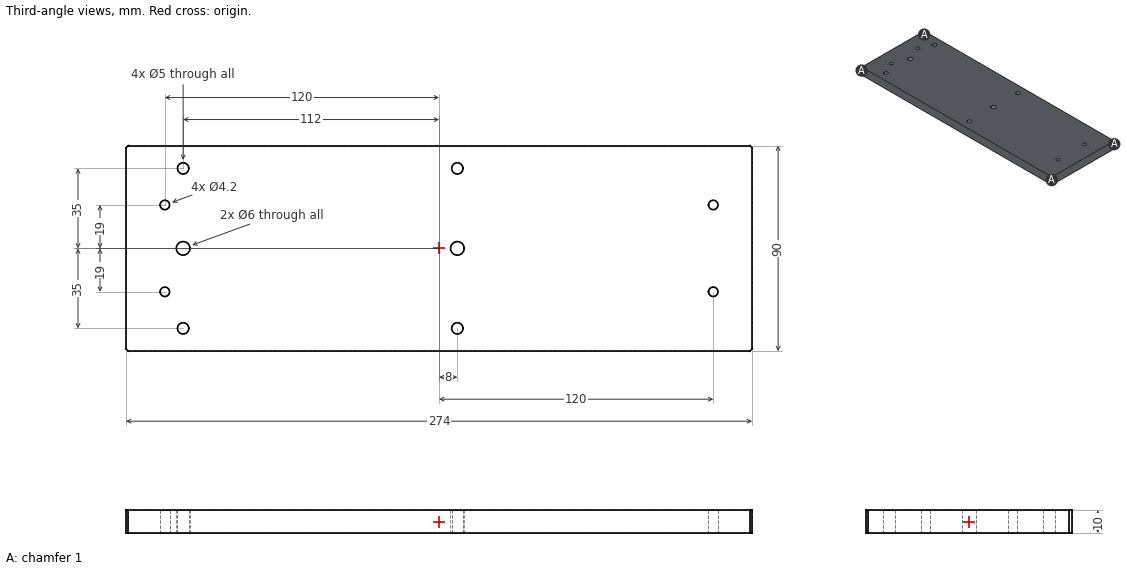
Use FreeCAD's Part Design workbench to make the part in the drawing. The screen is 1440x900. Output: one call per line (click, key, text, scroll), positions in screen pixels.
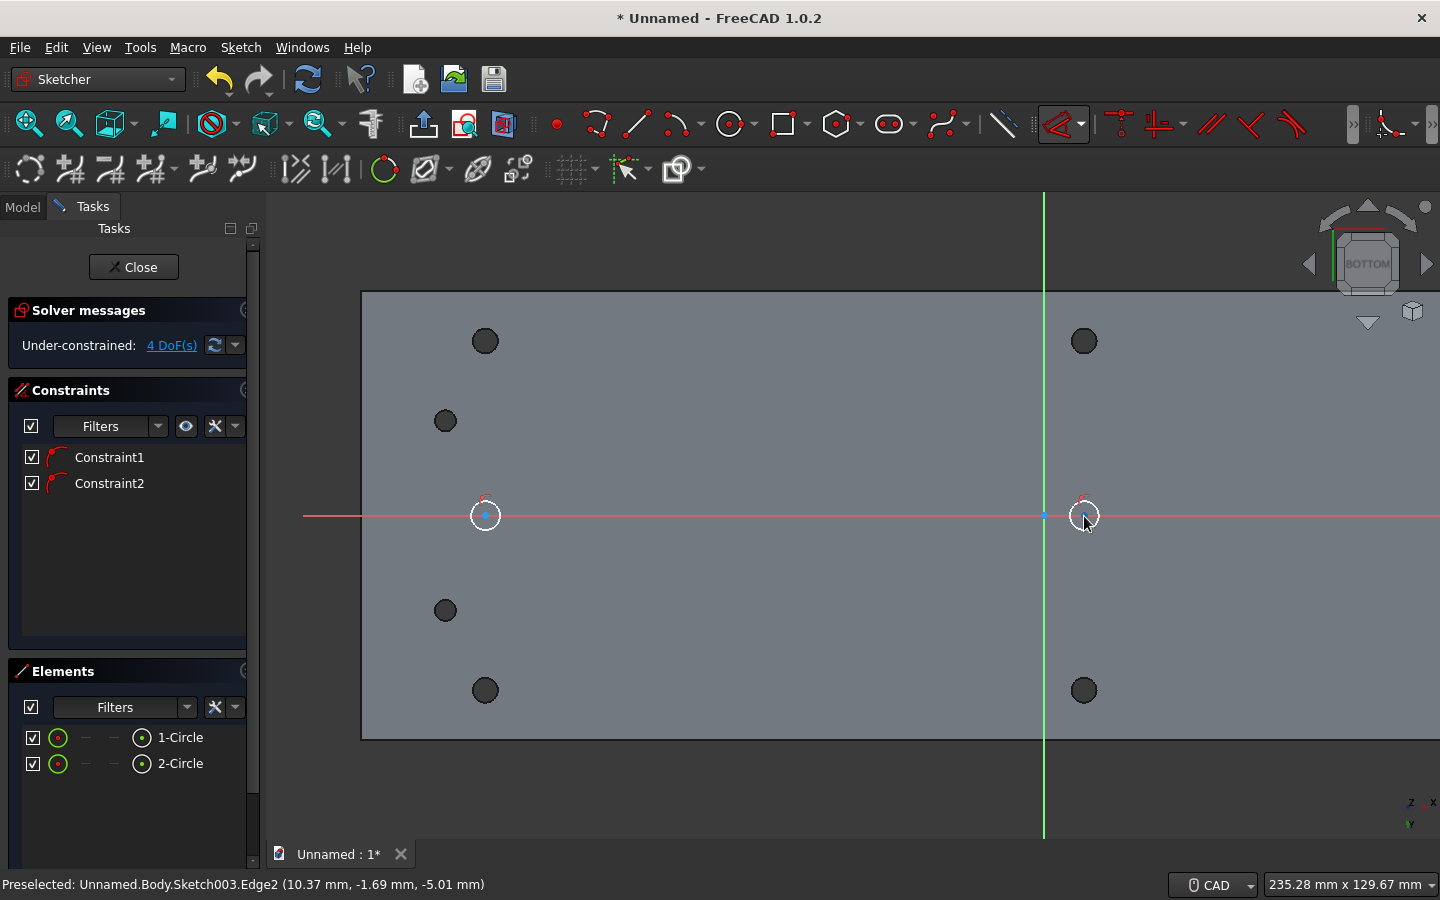
scroll(496, 505, up, 2)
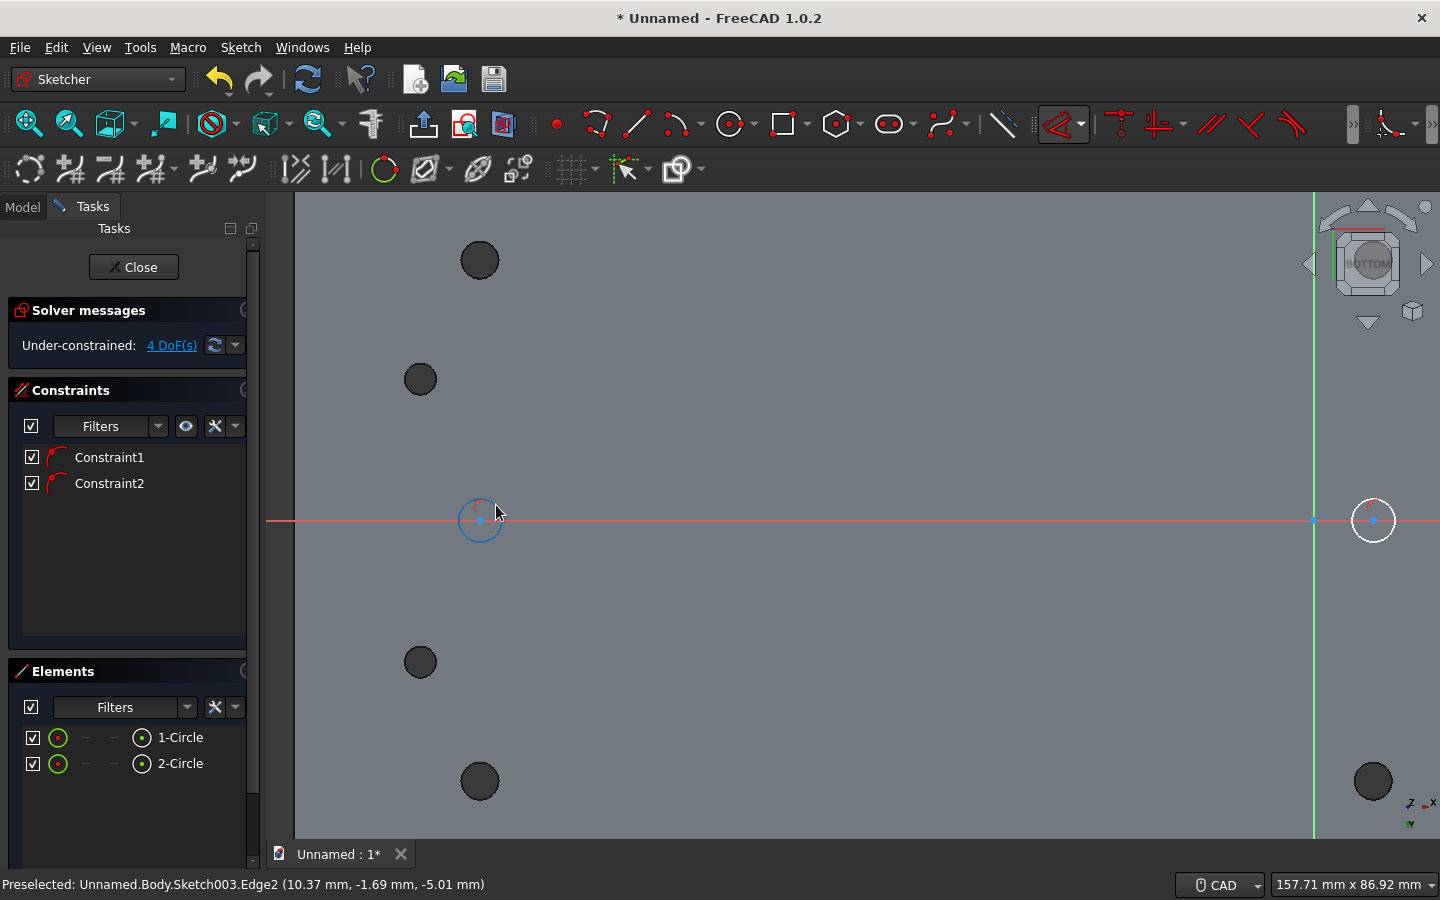
click(495, 505)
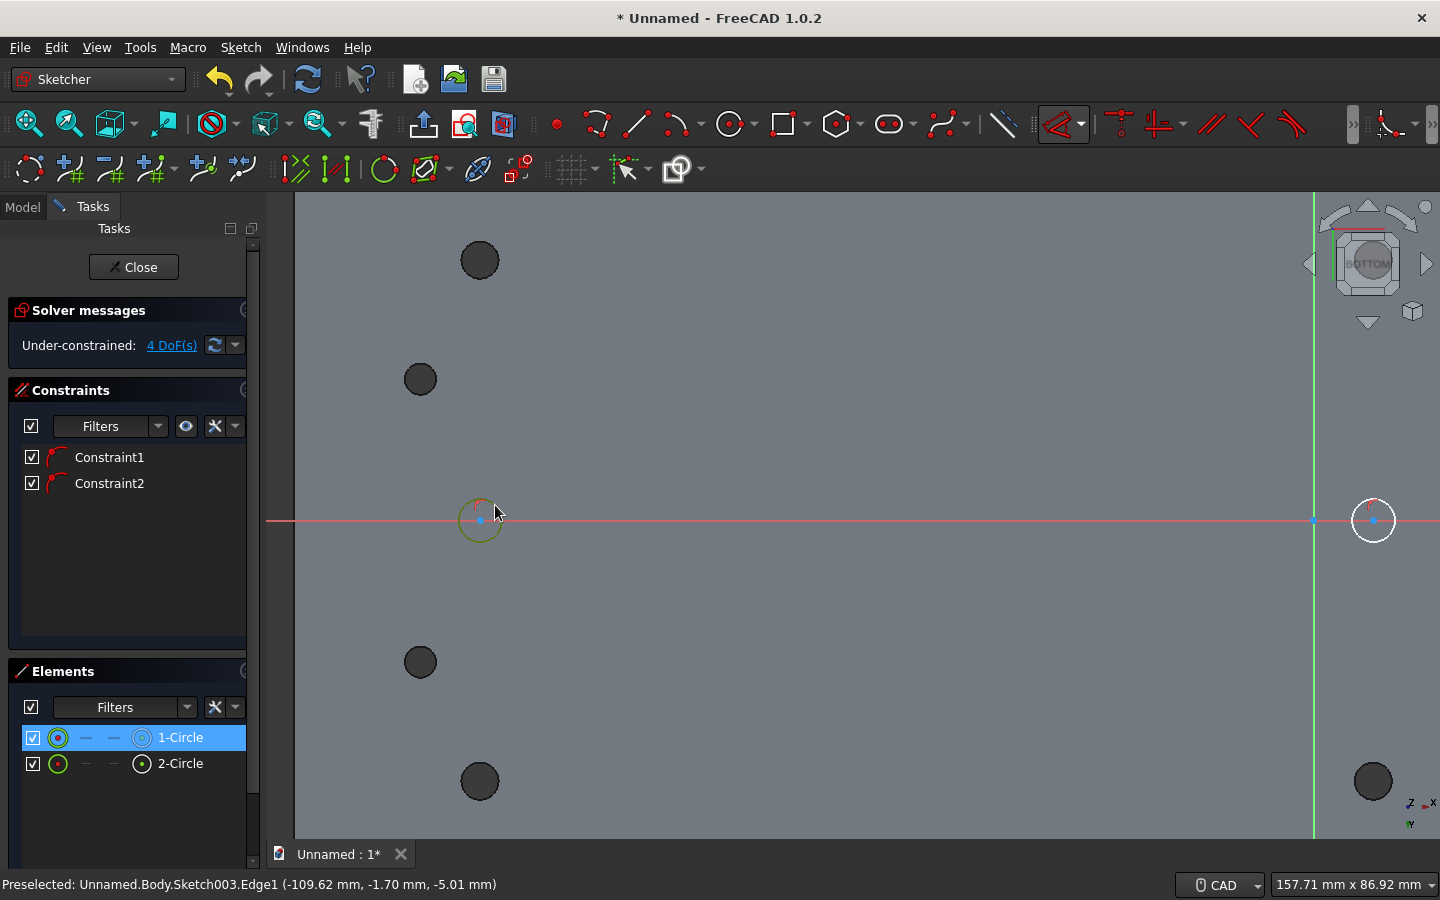
scroll(496, 505, down, 2)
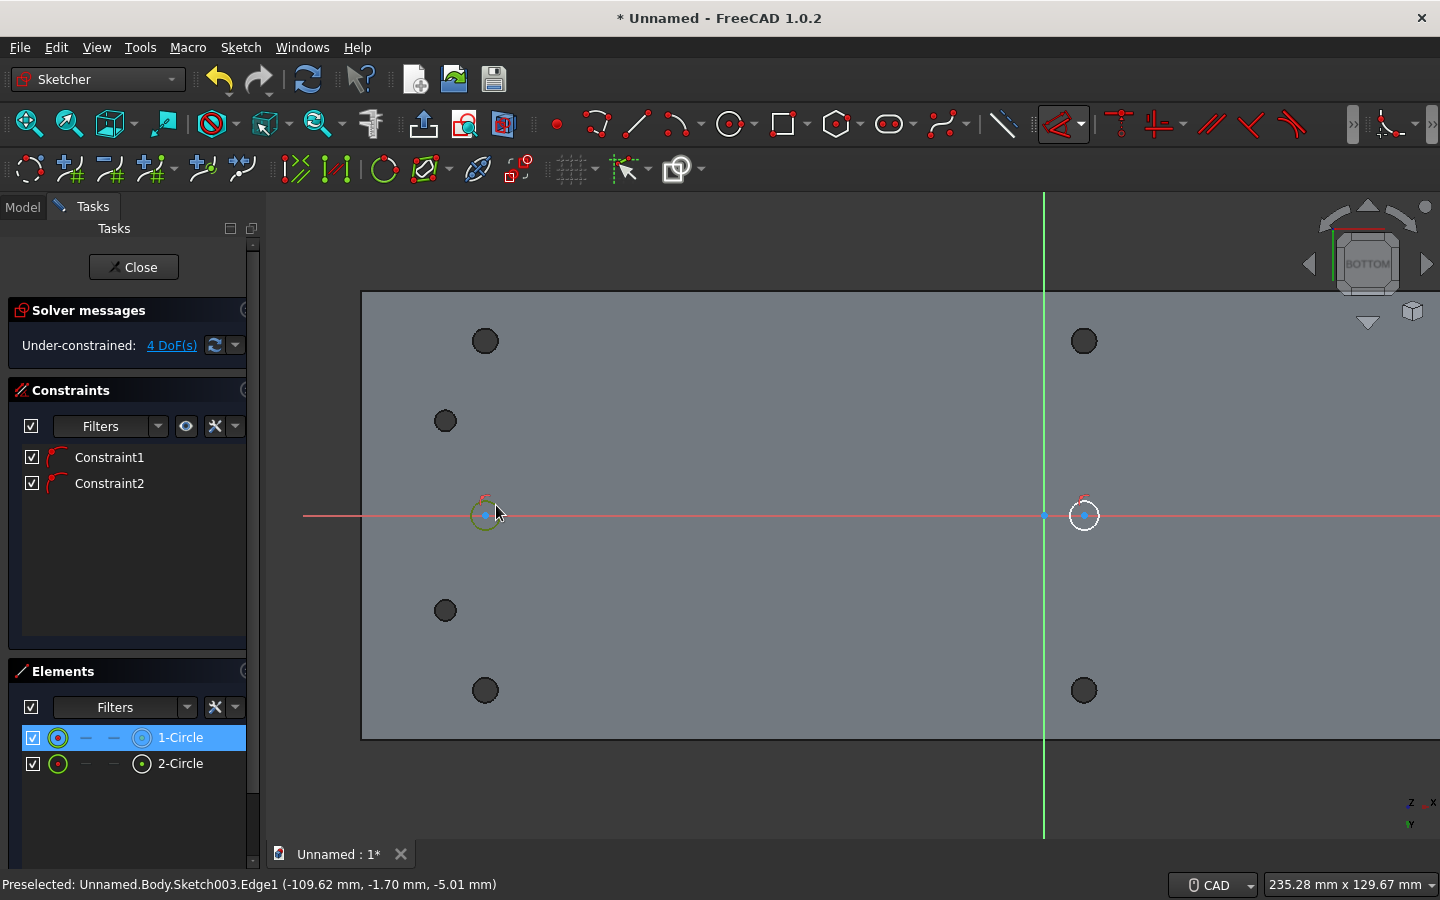
scroll(1094, 505, up, 2)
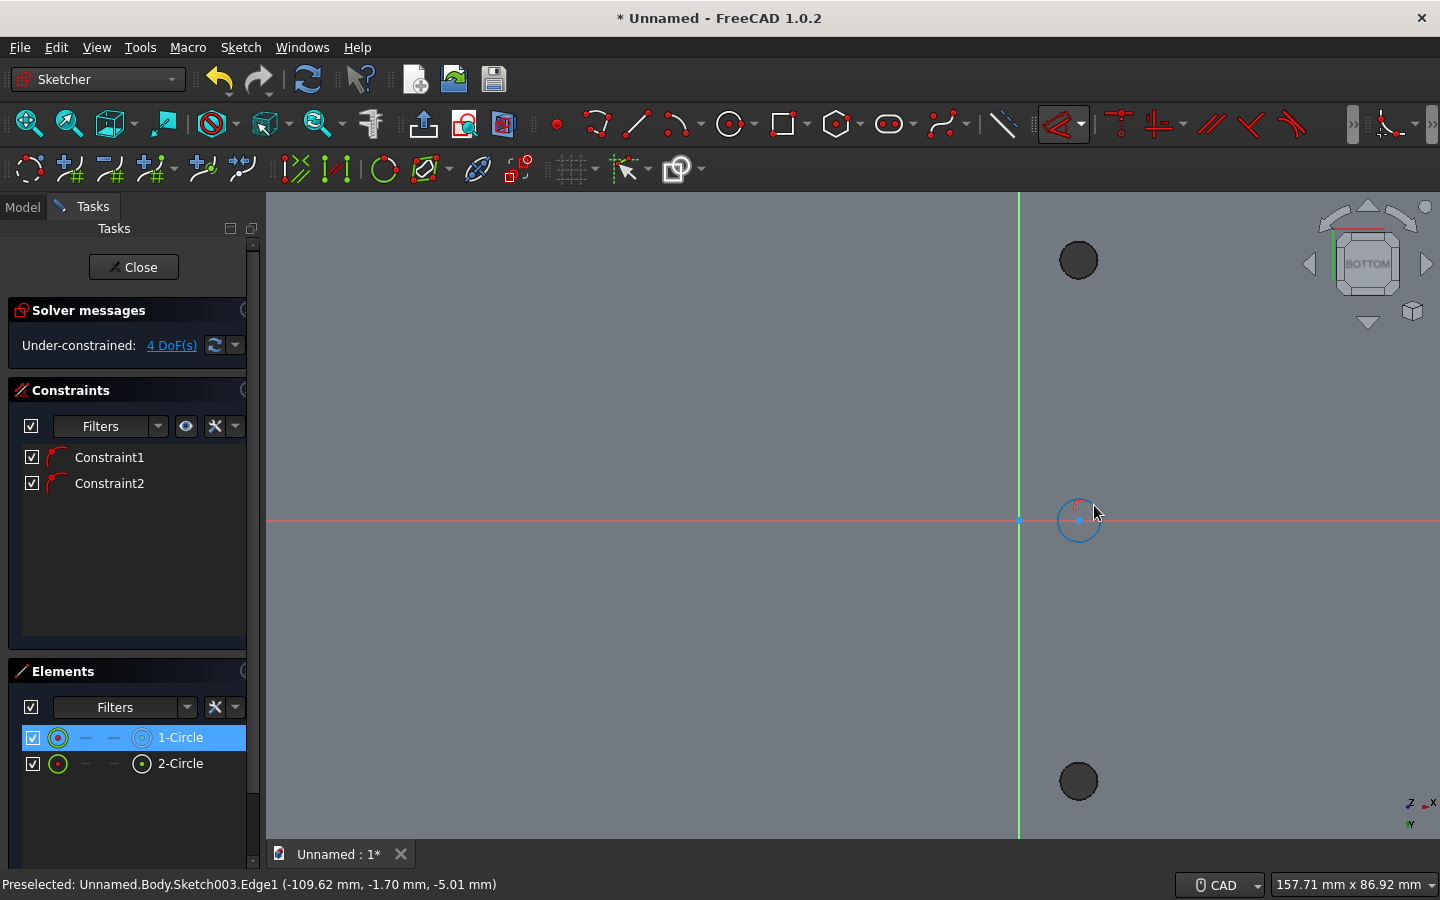
click(1094, 505)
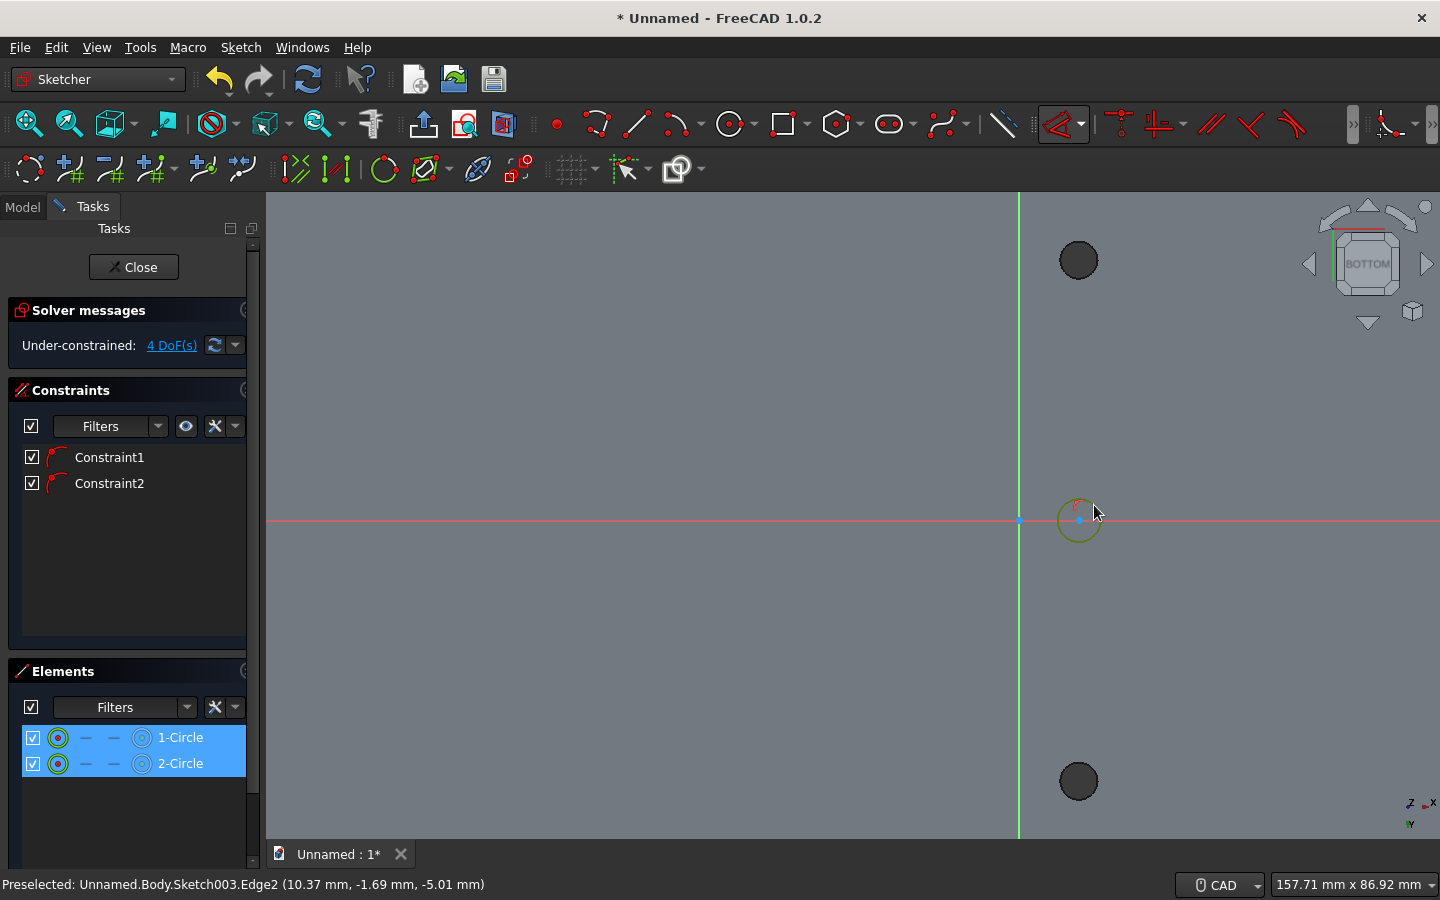
key(e)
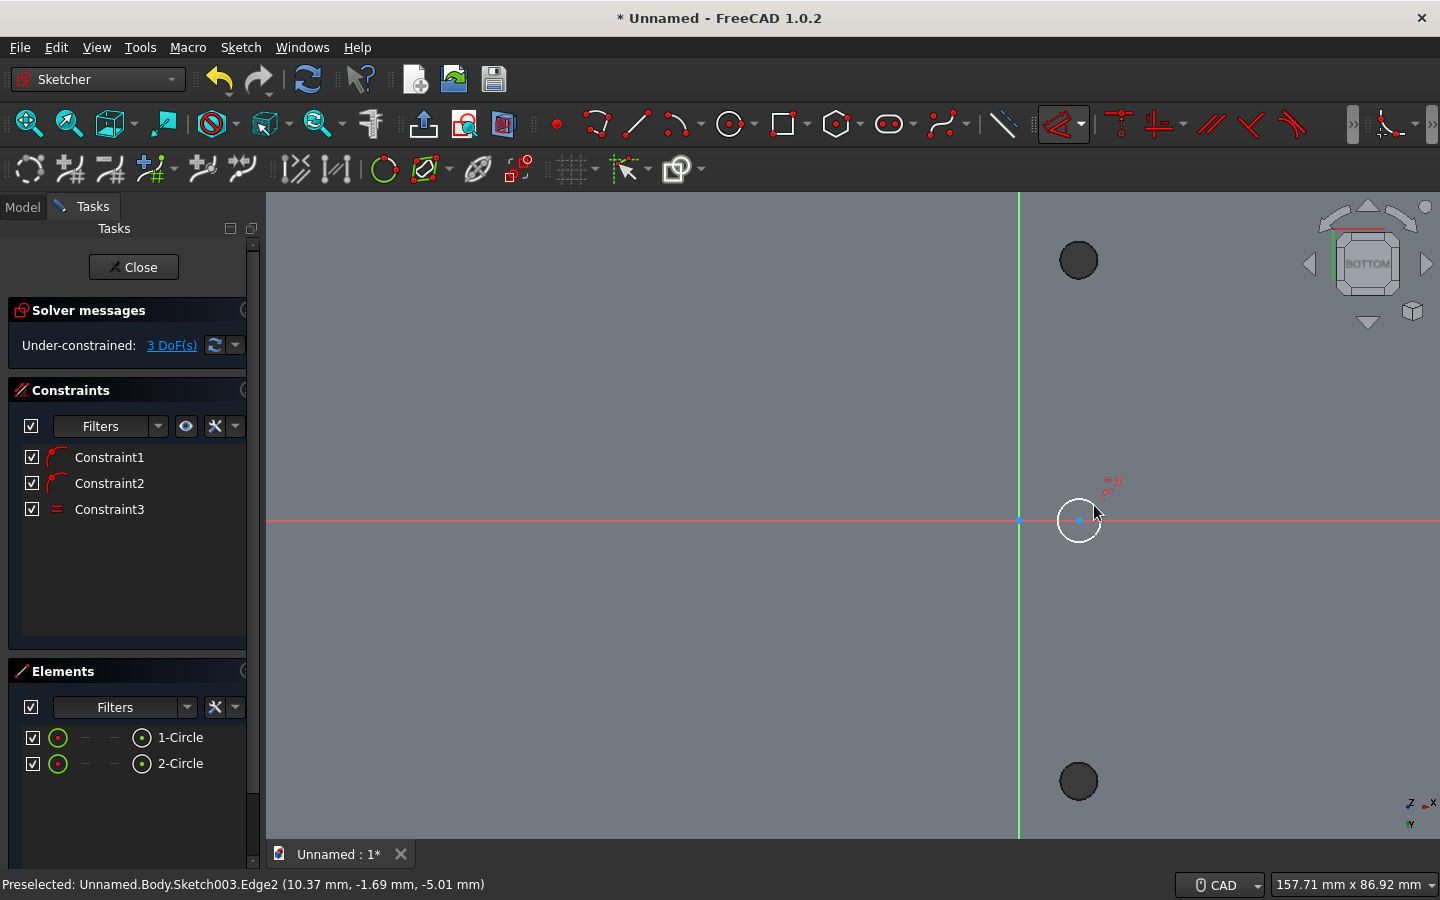
scroll(1094, 505, down, 2)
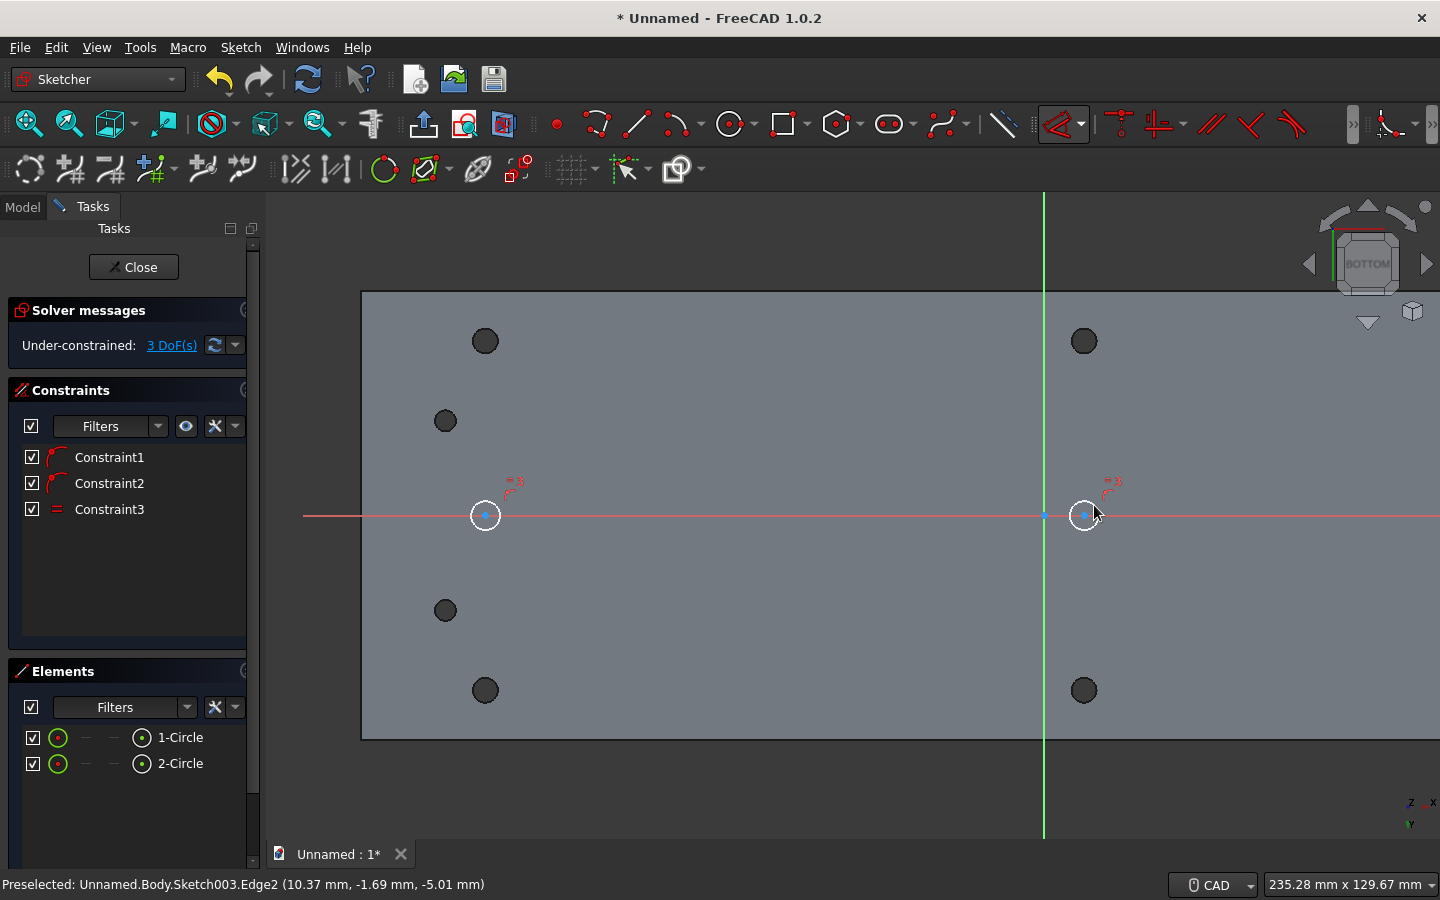
scroll(496, 505, up, 2)